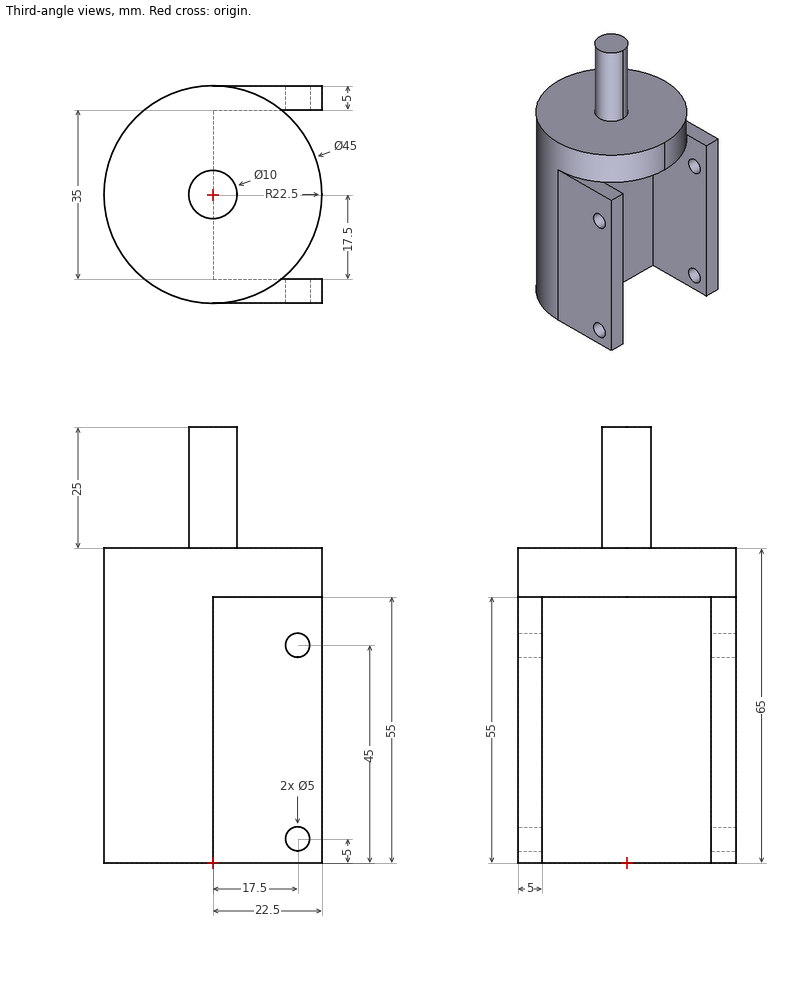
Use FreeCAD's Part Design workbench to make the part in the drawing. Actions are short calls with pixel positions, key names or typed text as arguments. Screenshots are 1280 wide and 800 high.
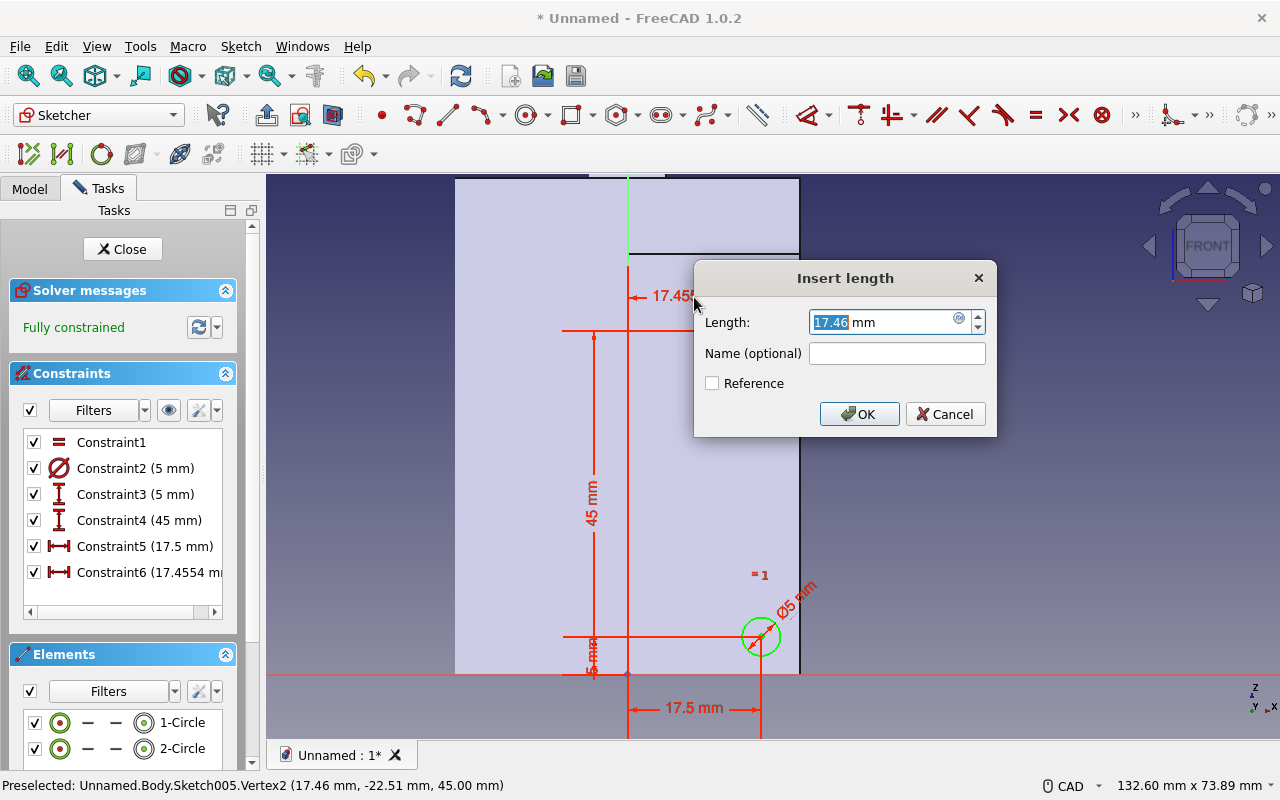
text(17.5)
key(Return)
key(Escape)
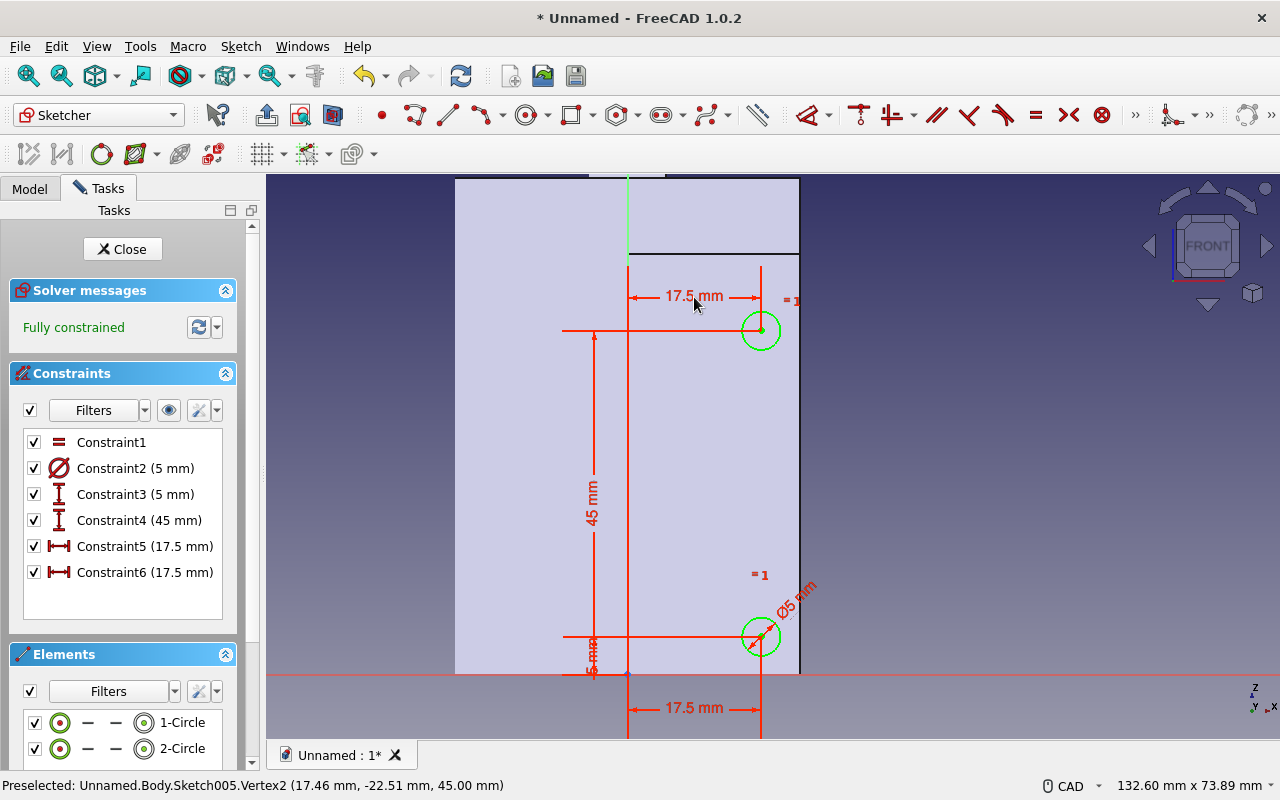
click(123, 249)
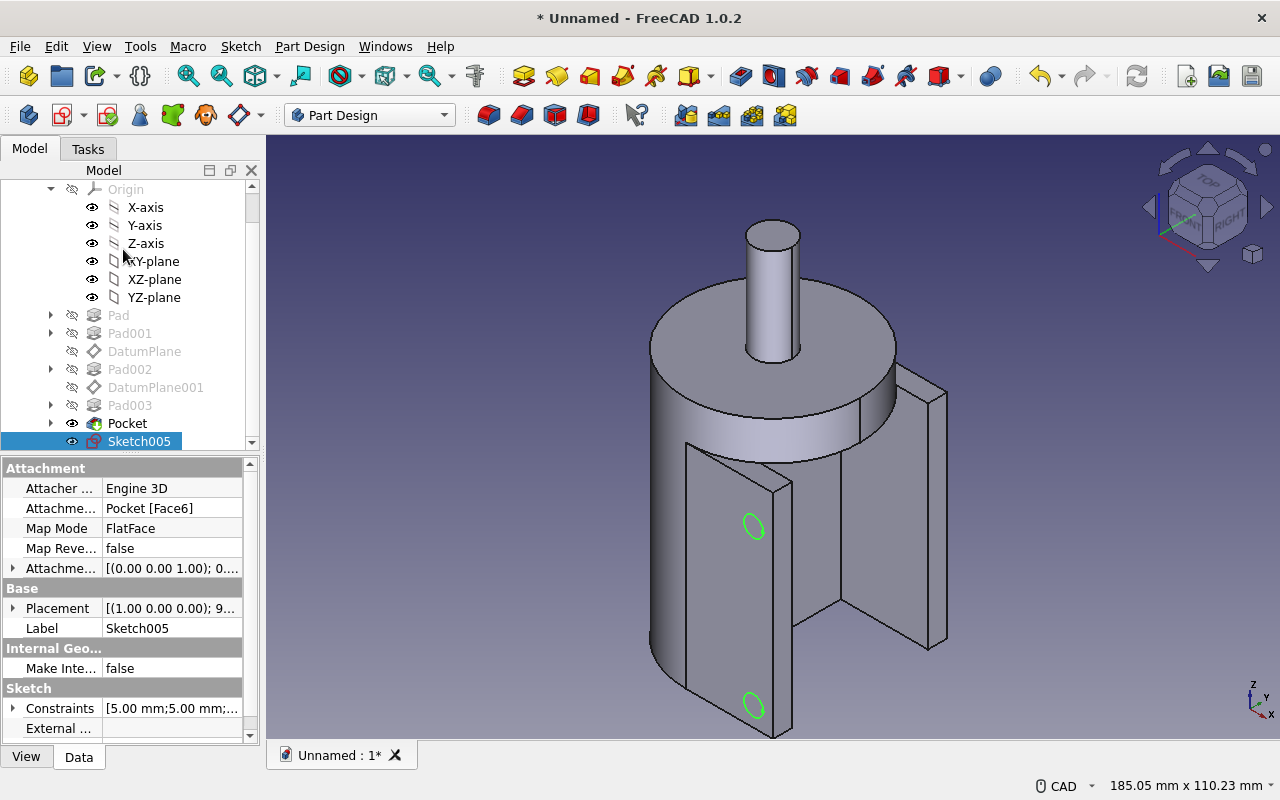
click(741, 76)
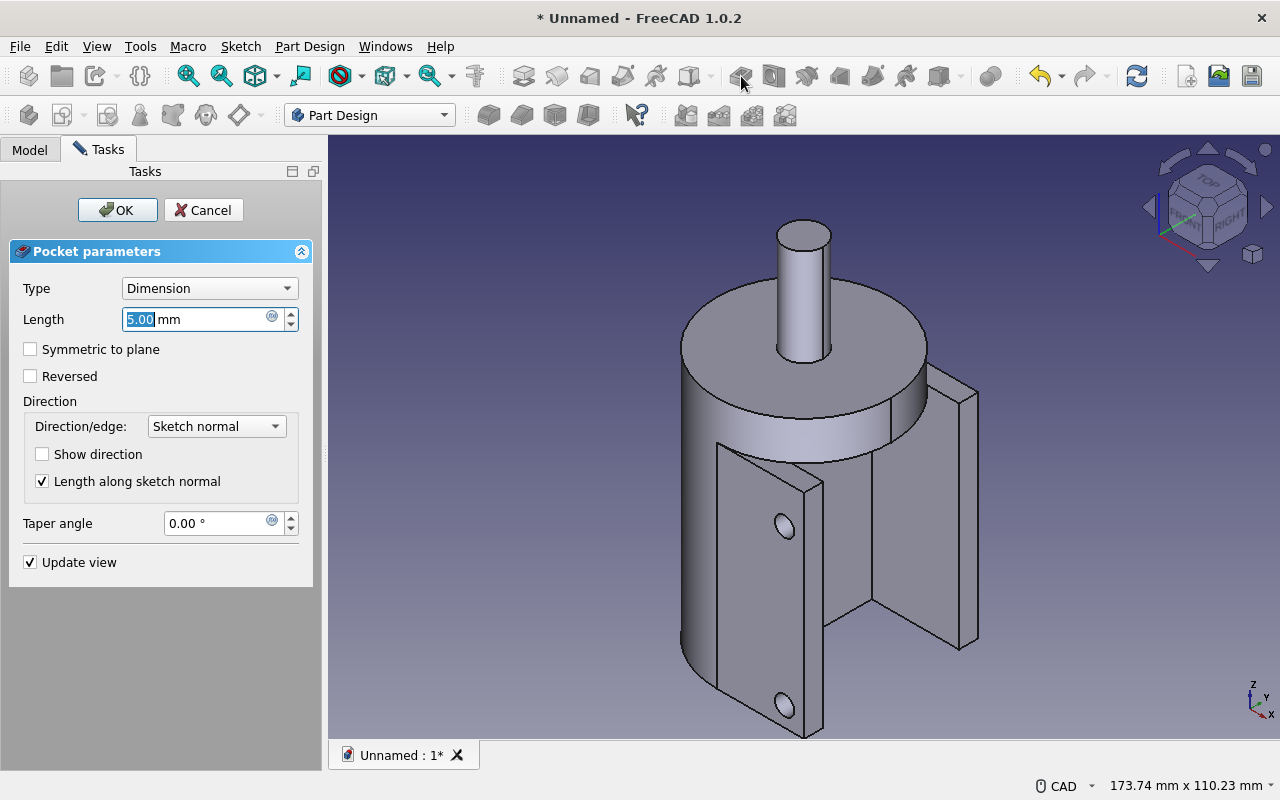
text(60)
key(Tab)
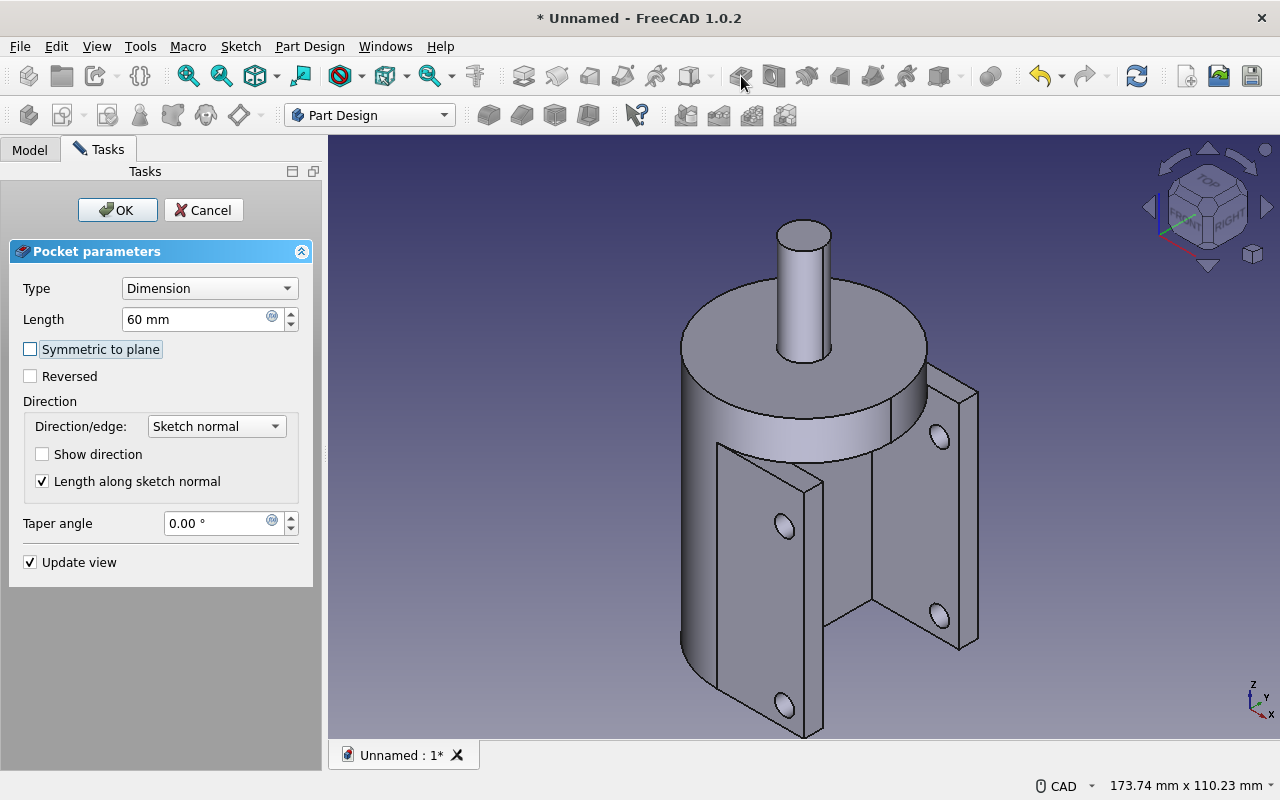
click(118, 210)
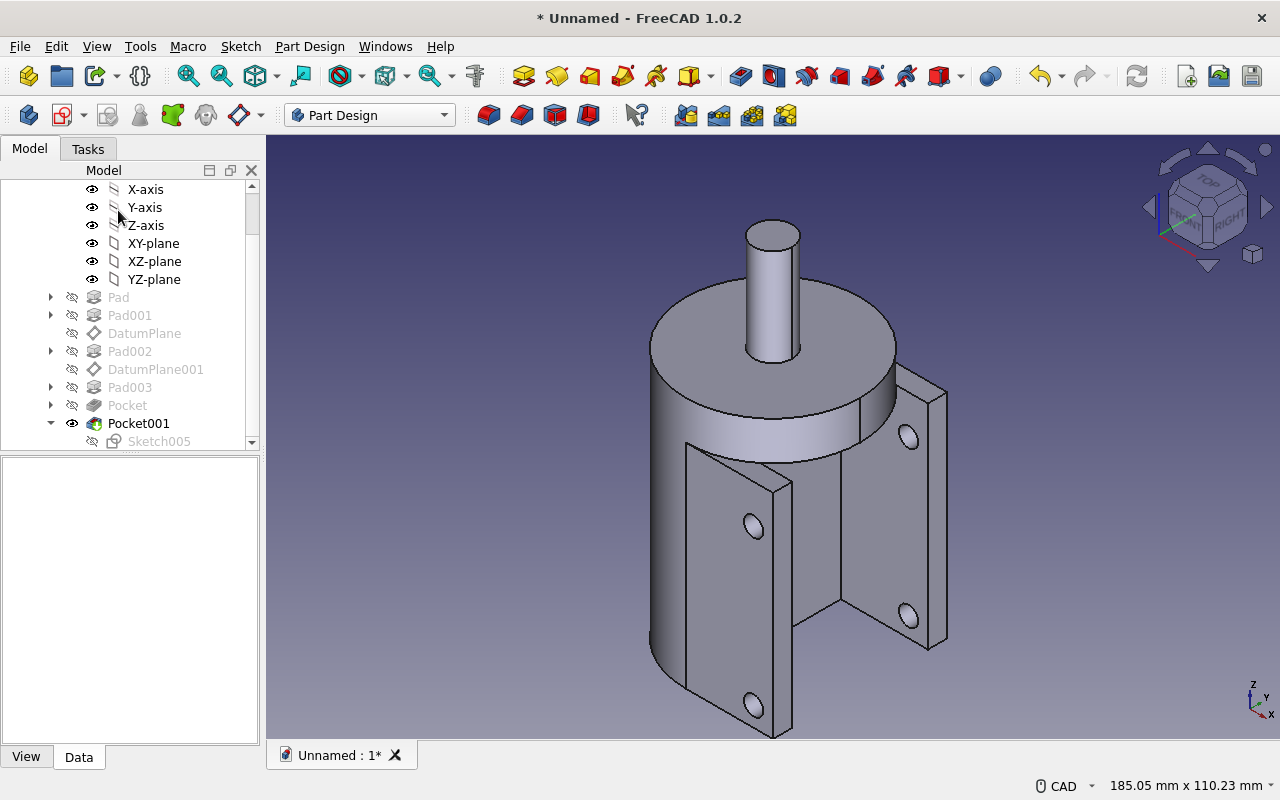
click(189, 76)